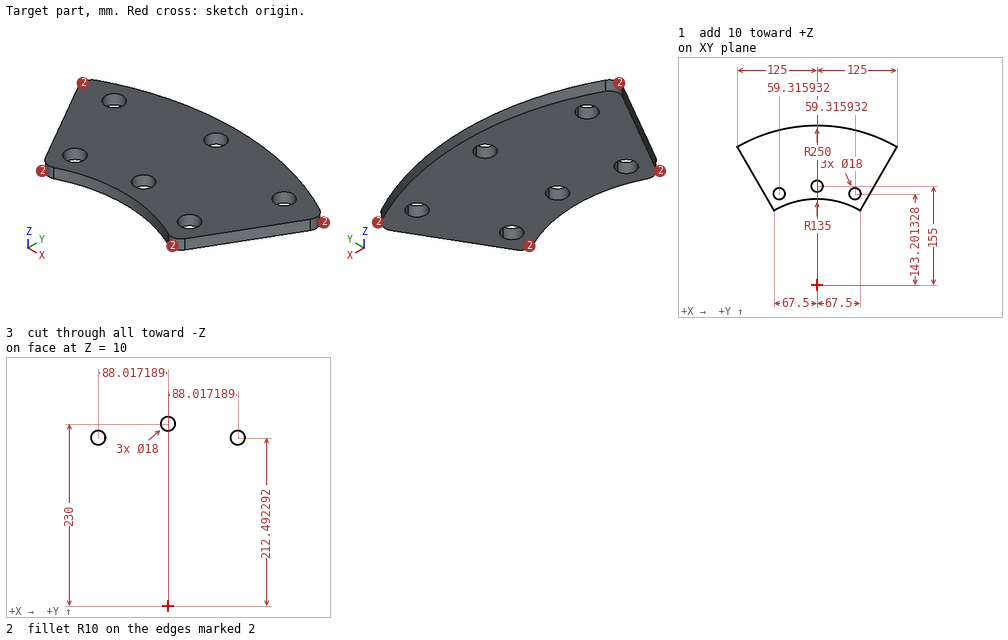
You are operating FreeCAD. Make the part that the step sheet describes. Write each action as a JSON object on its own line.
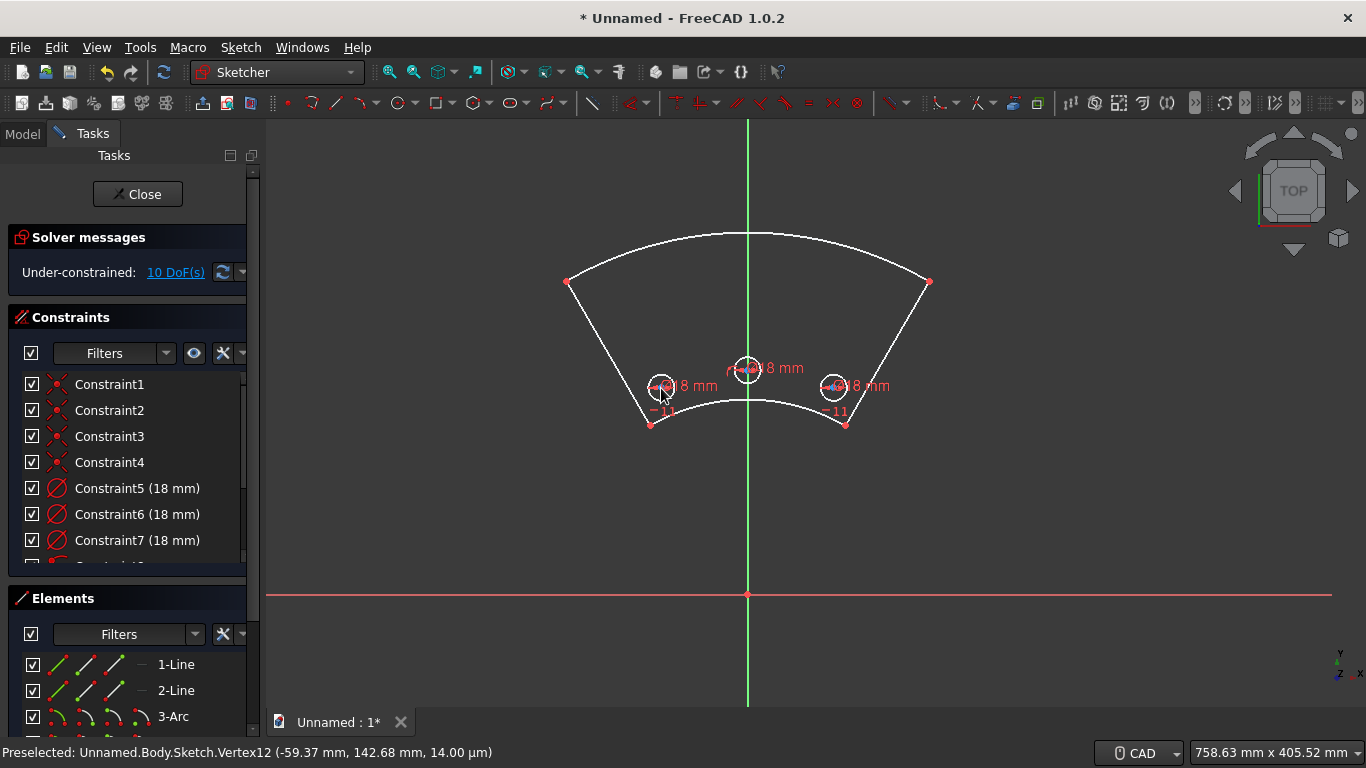
{"action": "left_click", "coordinate": [788, 404]}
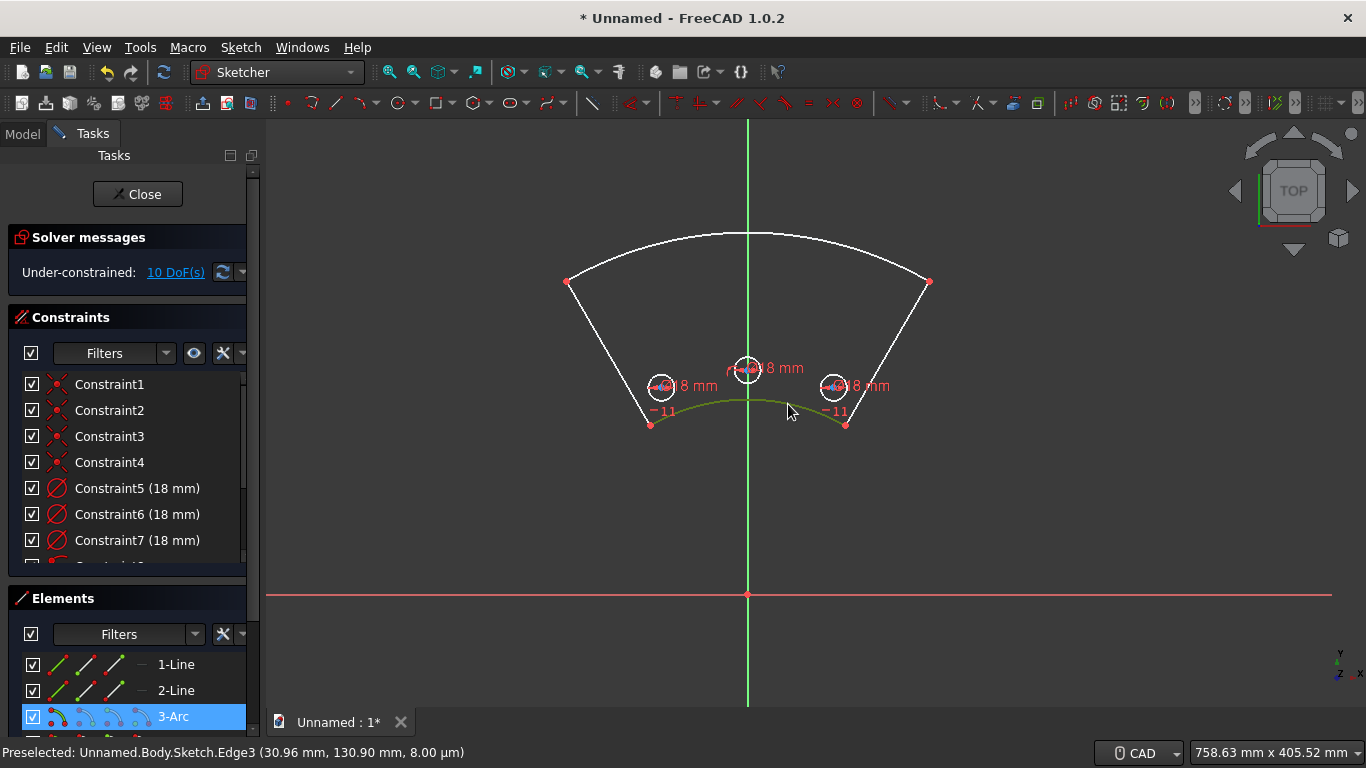
{"action": "key", "text": "k r"}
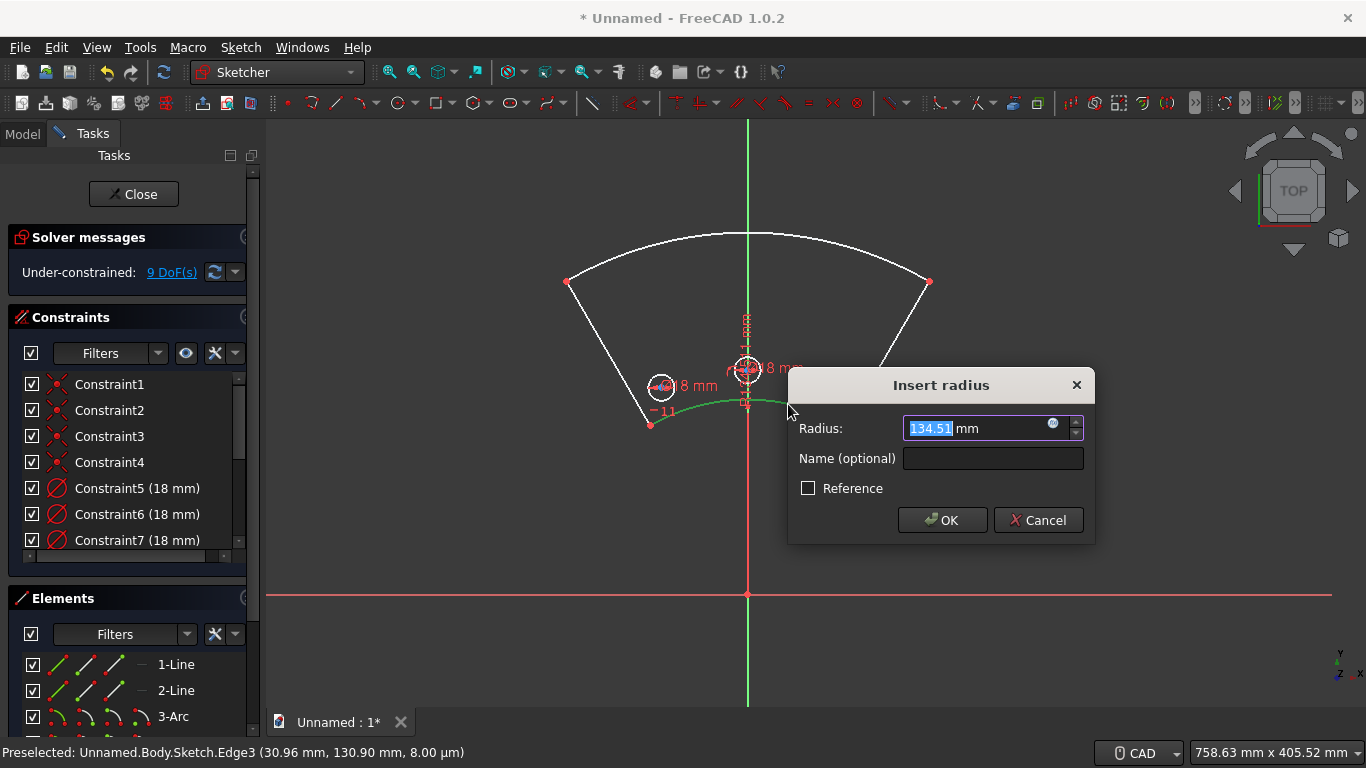
{"action": "type", "text": "135"}
{"action": "key", "text": "Return"}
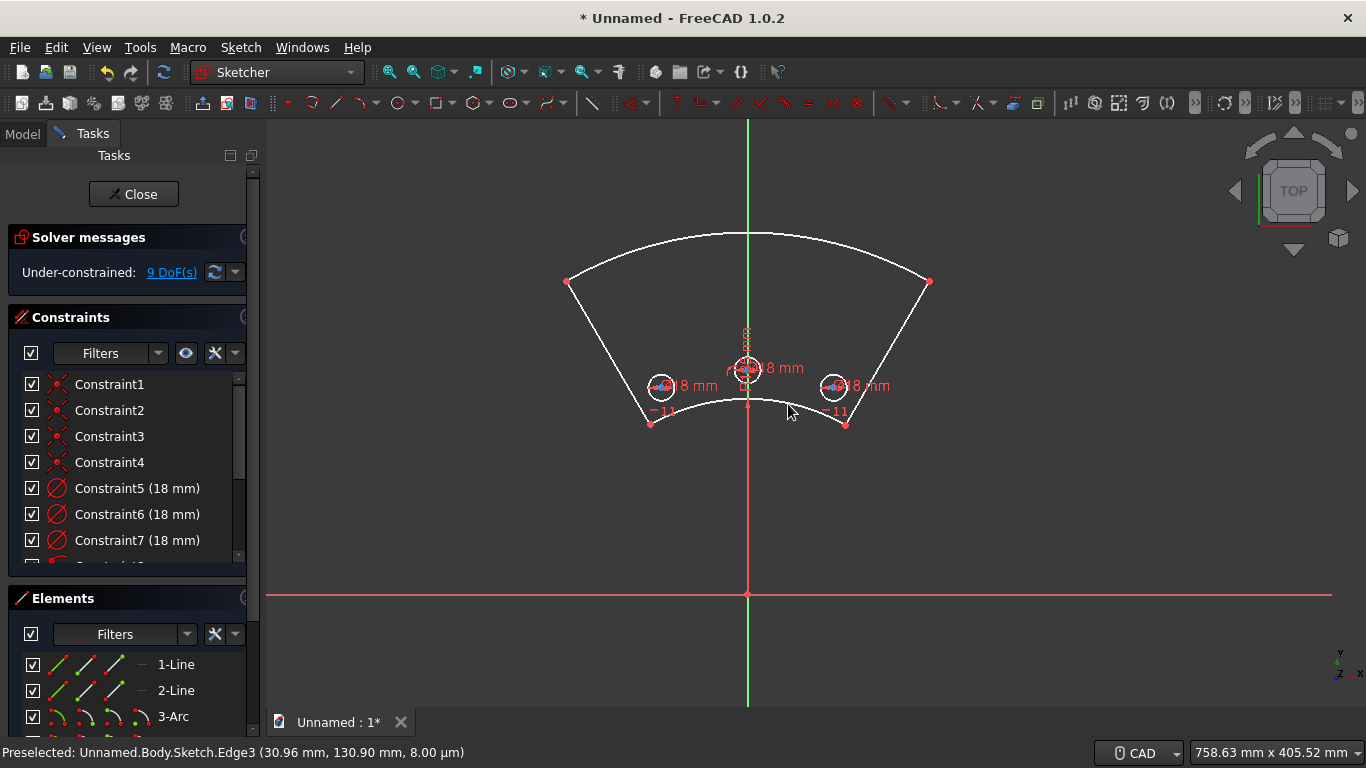
{"action": "left_click", "coordinate": [823, 241]}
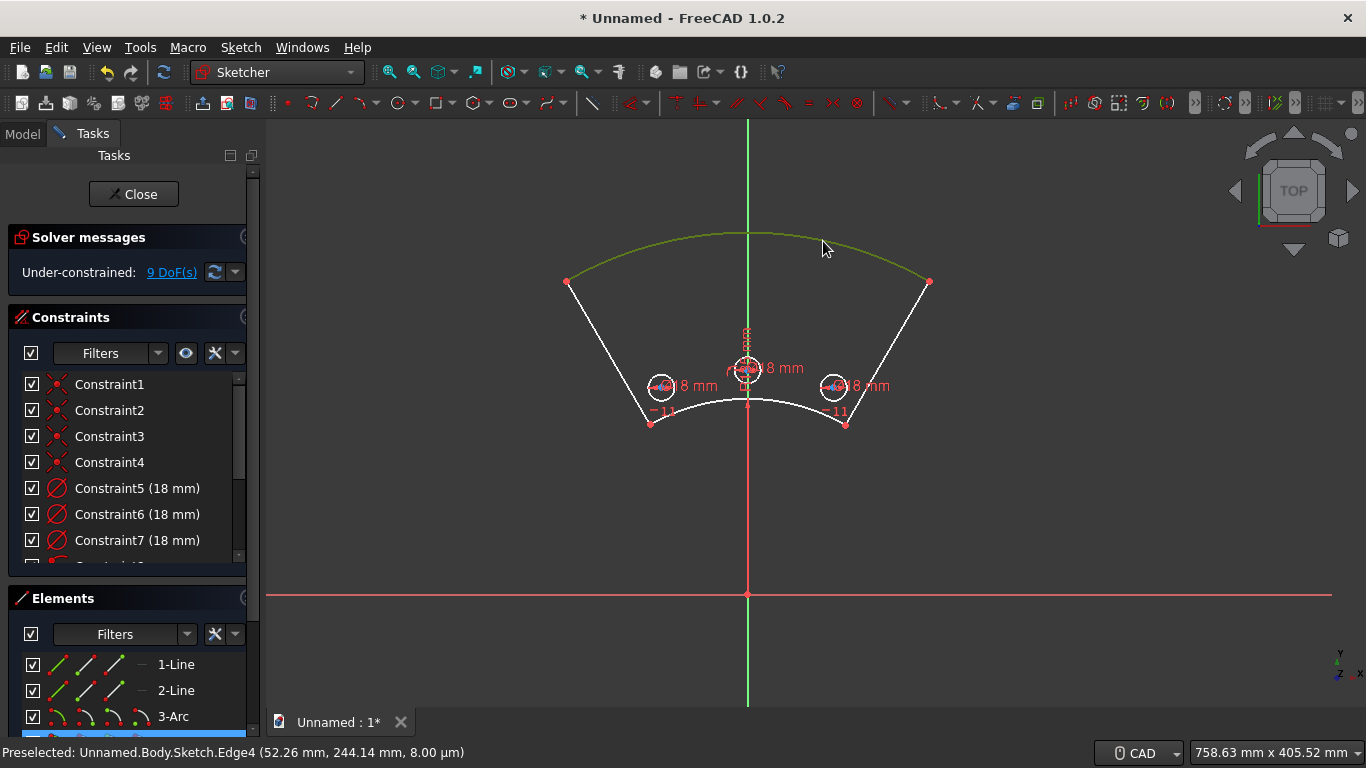
{"action": "key", "text": "k r"}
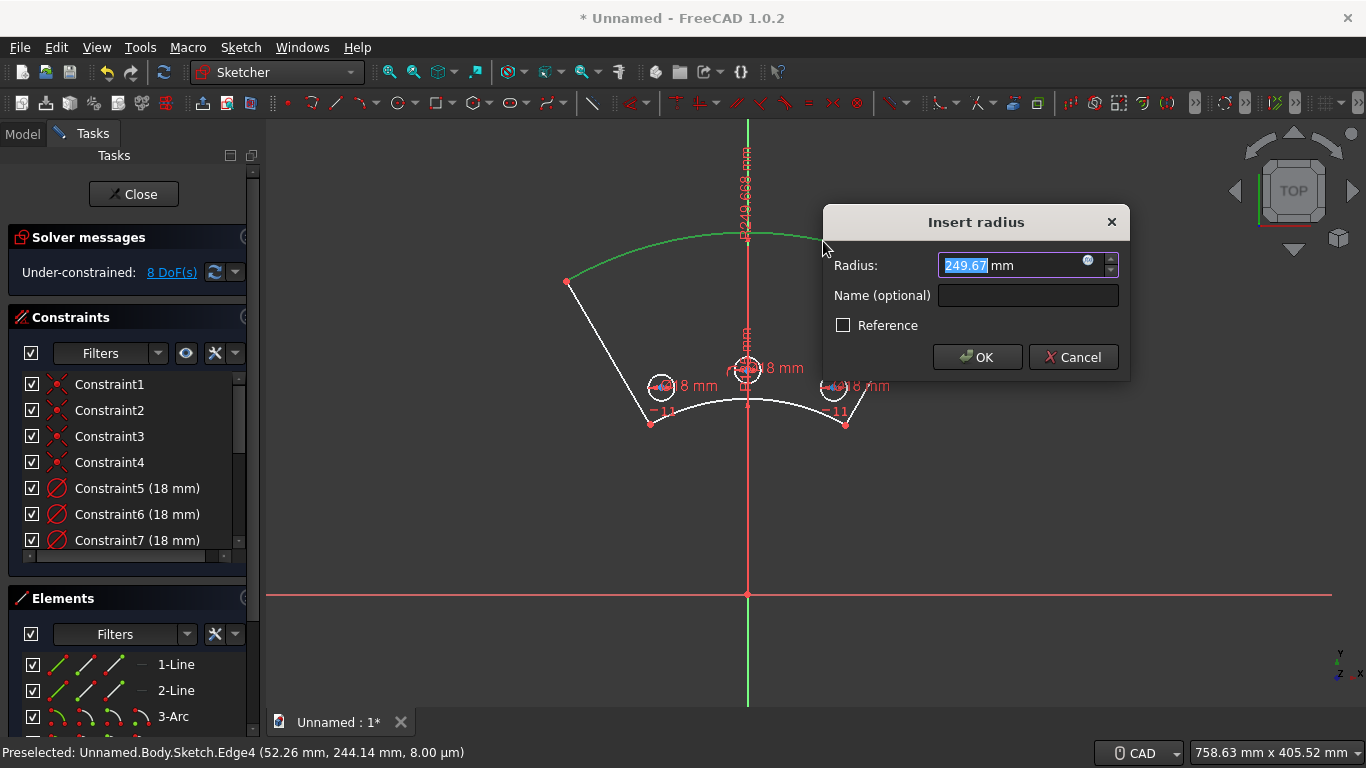
{"action": "type", "text": "250"}
{"action": "key", "text": "Return"}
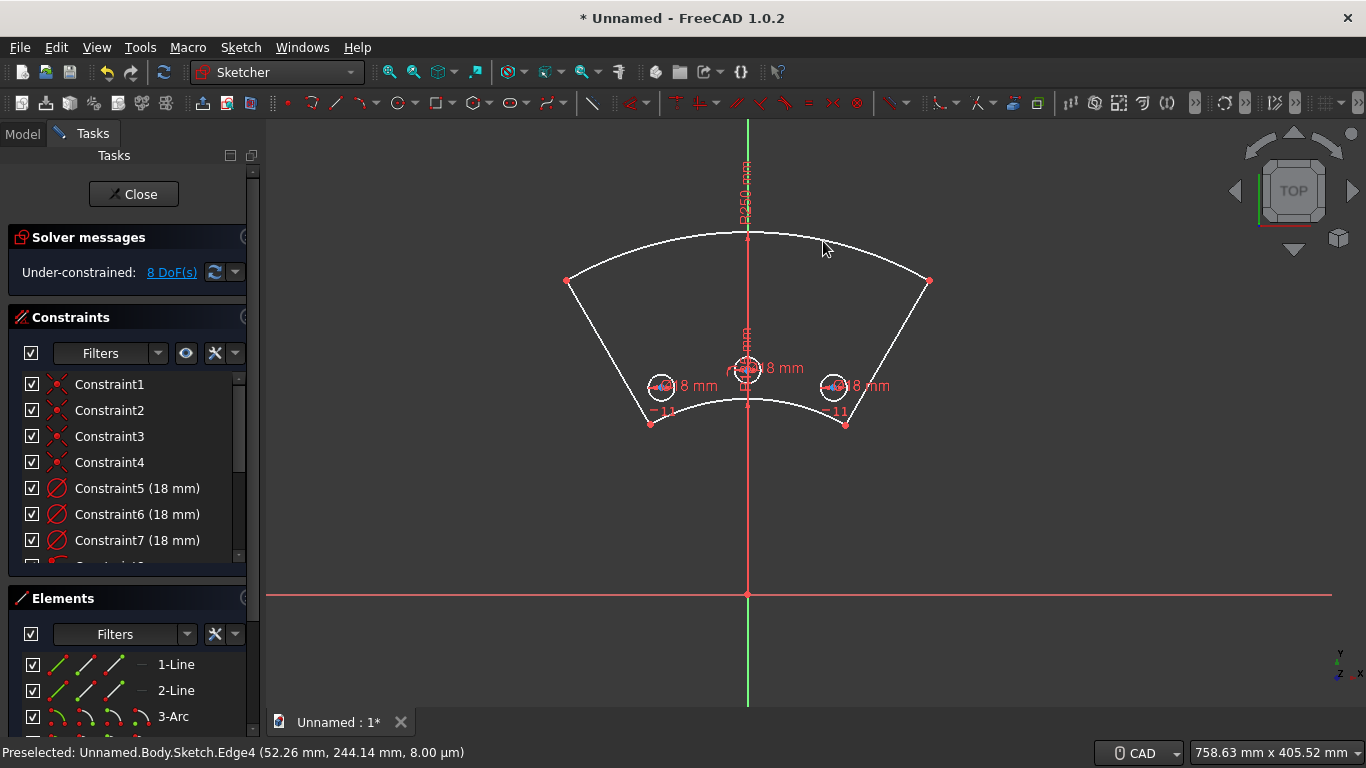
{"action": "left_click", "coordinate": [748, 370]}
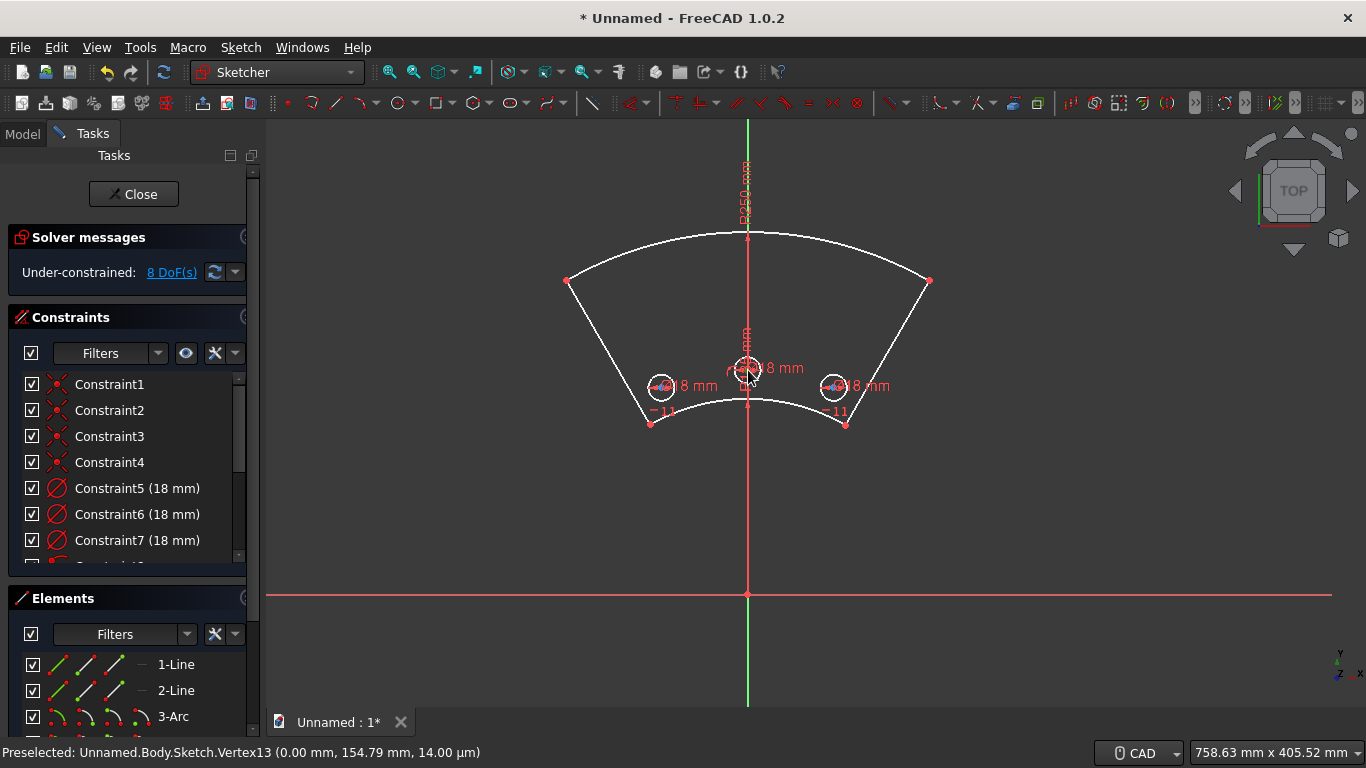
{"action": "left_click", "coordinate": [648, 104]}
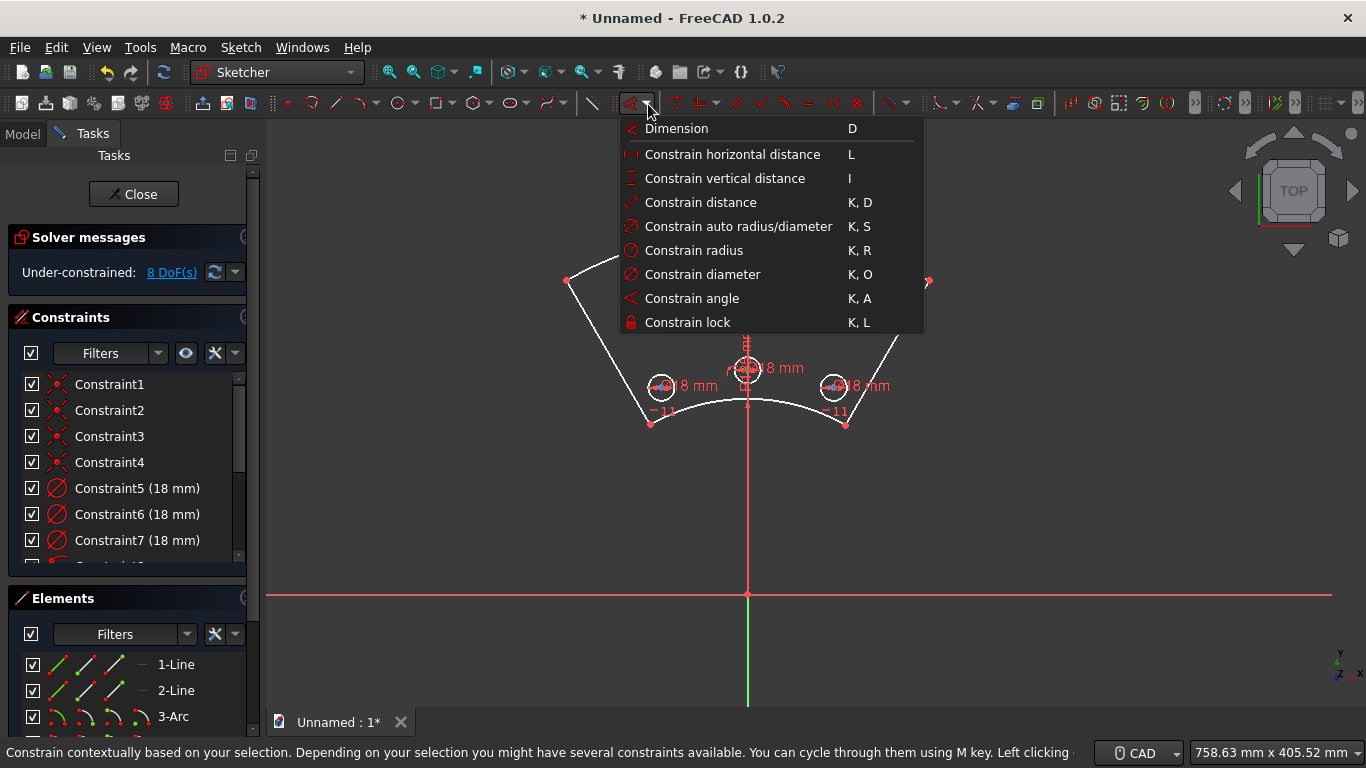
{"action": "left_click", "coordinate": [772, 178]}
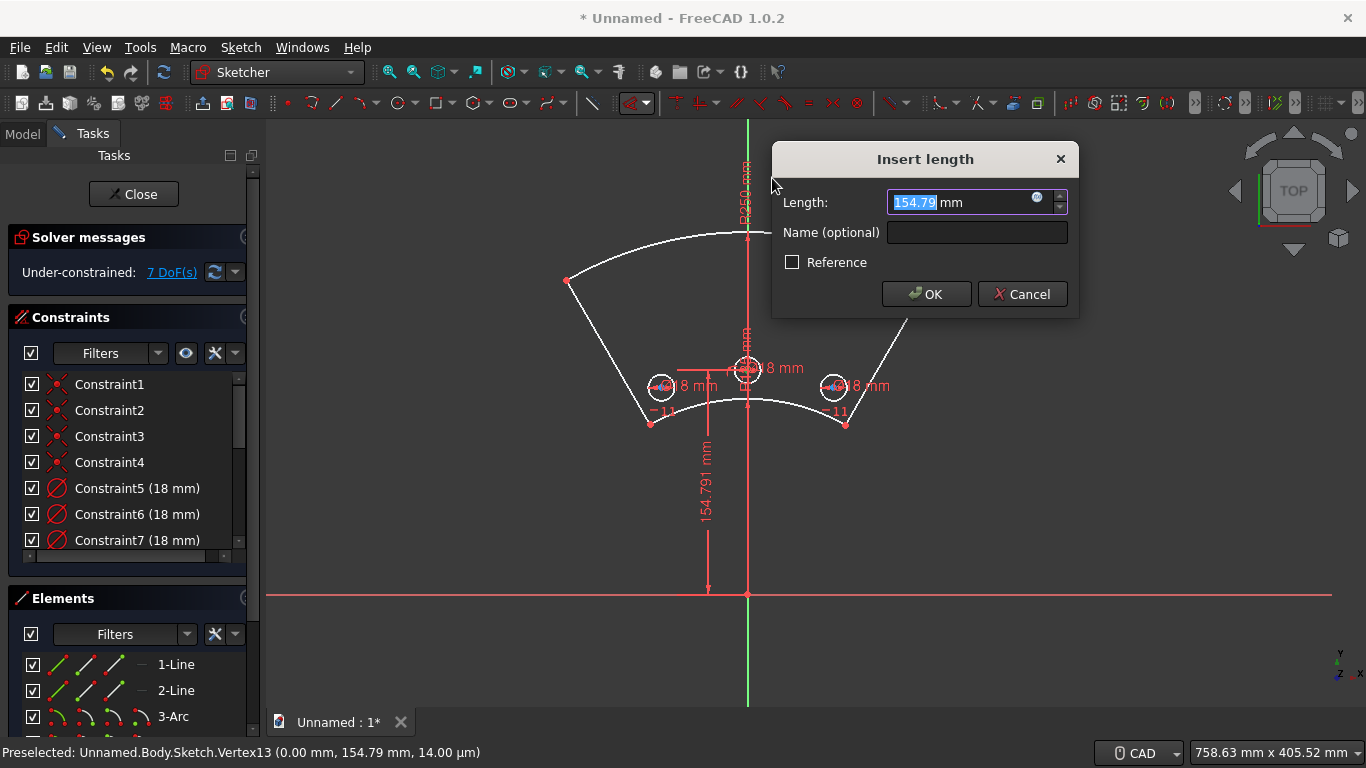
{"action": "type", "text": "155"}
{"action": "key", "text": "Return"}